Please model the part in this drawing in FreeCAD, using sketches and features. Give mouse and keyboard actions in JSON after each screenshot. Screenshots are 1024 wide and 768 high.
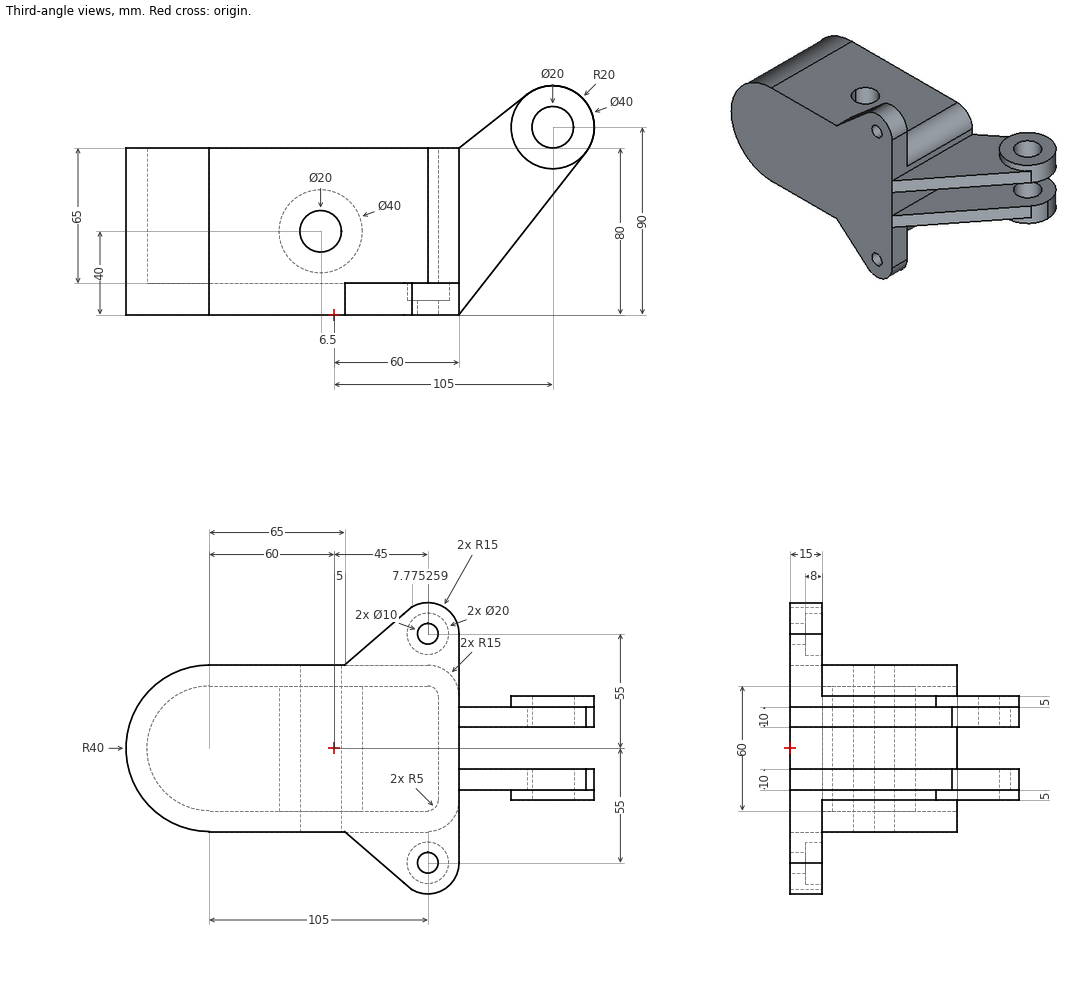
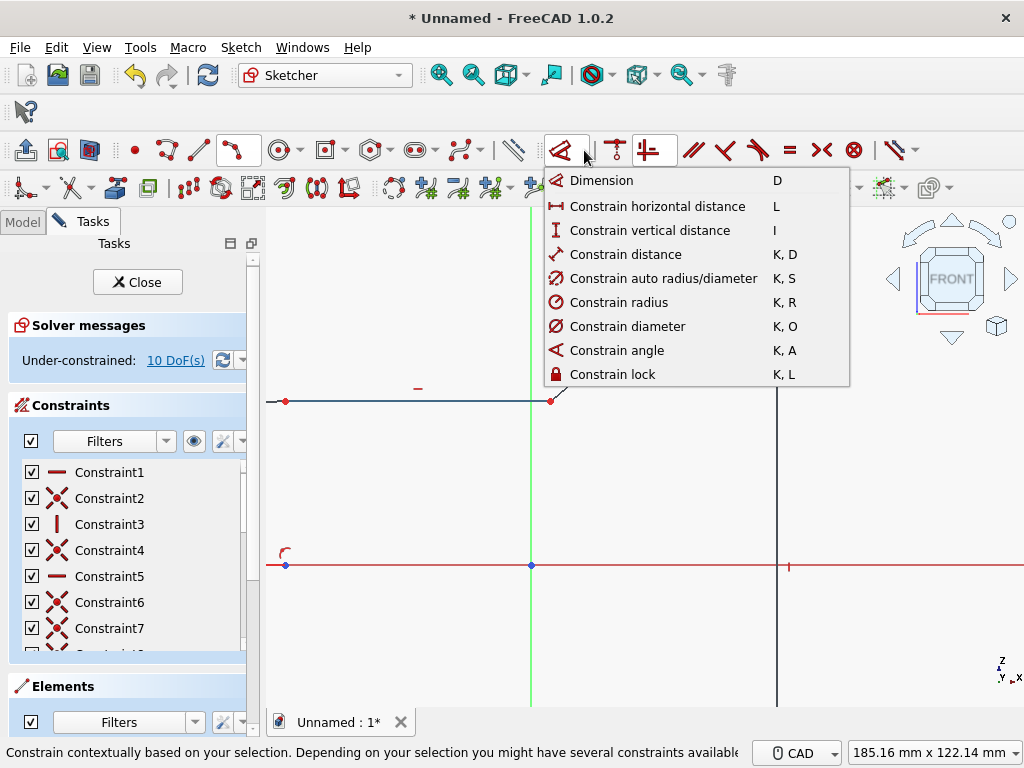
{"action": "left_click", "coordinate": [697, 206]}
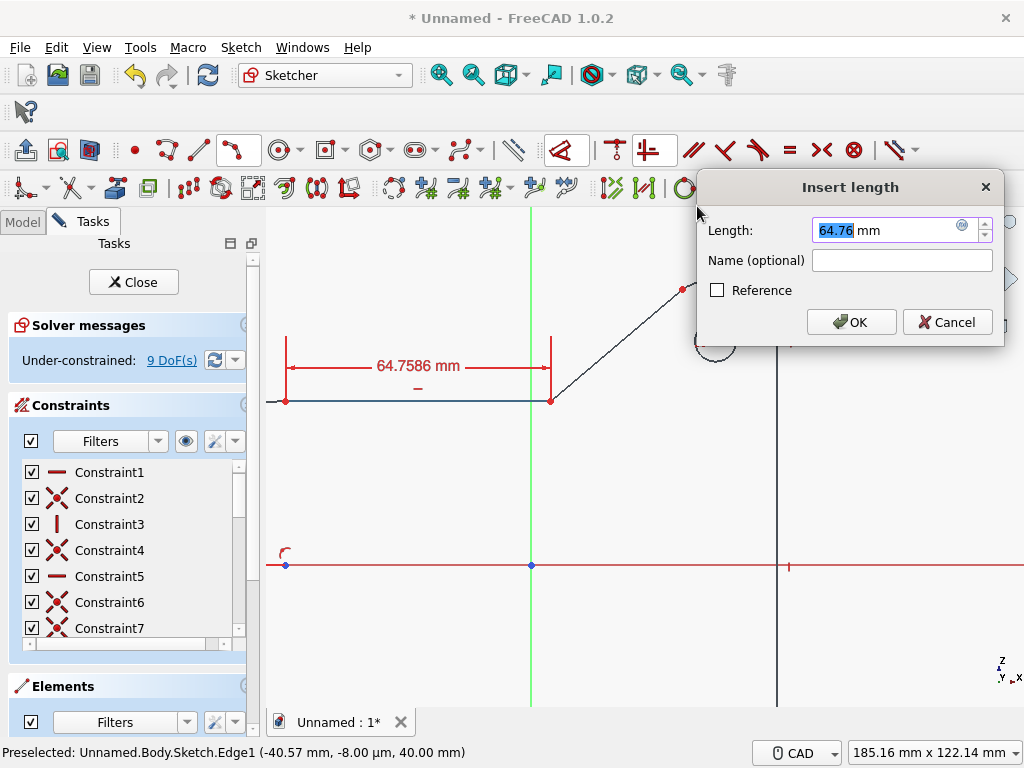
{"action": "type", "text": "65"}
{"action": "key", "text": "Return"}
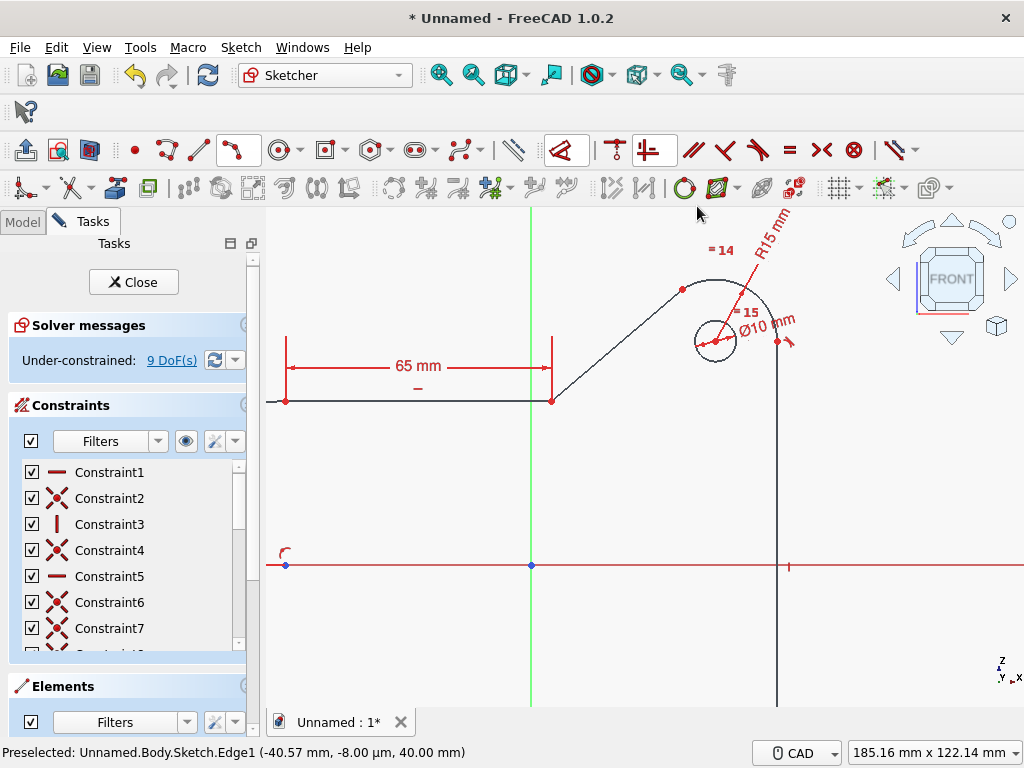
{"action": "scroll", "coordinate": [731, 326], "scroll_direction": "down", "scroll_amount": 3}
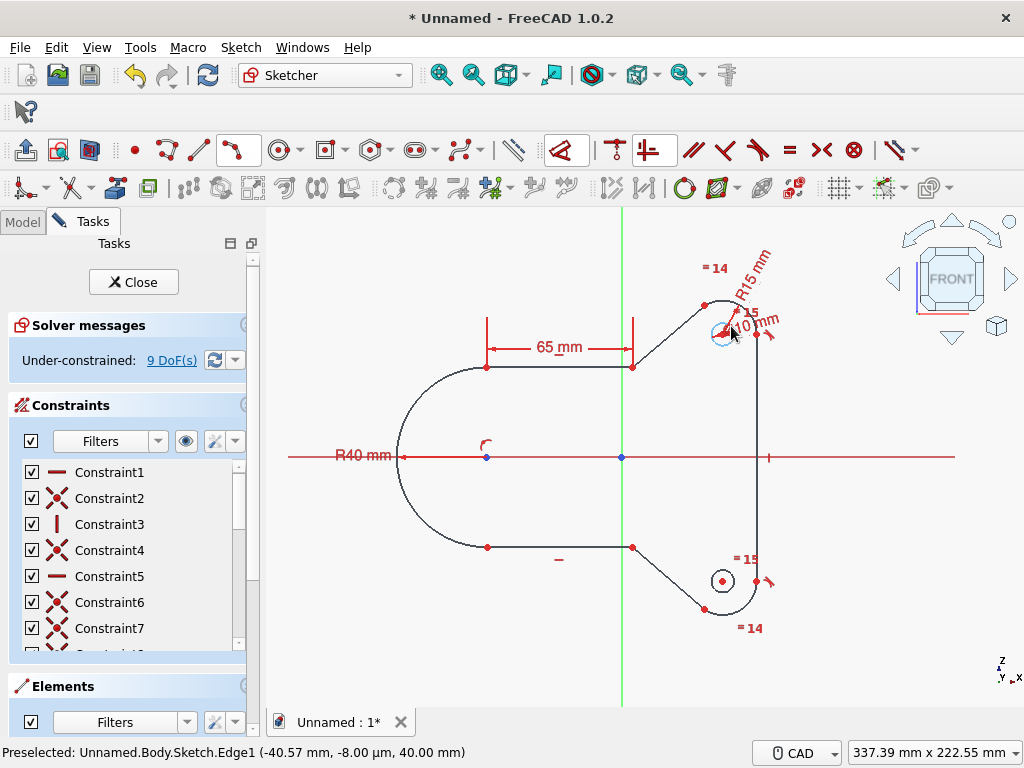
{"action": "left_click", "coordinate": [589, 547]}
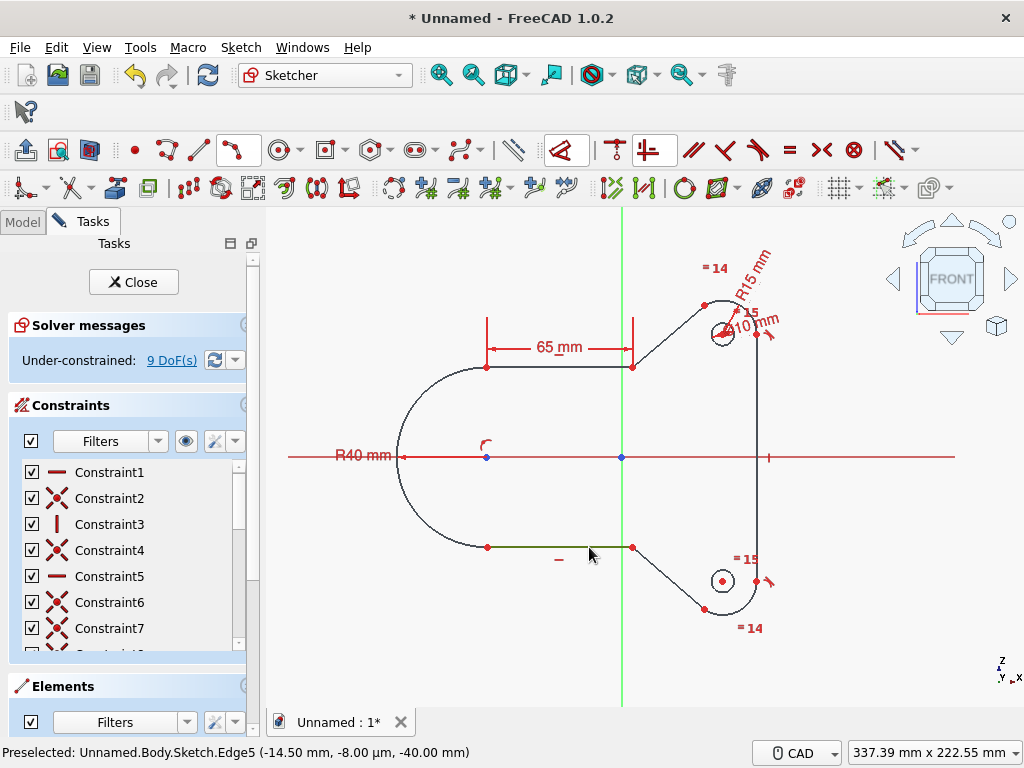
{"action": "key", "text": "l"}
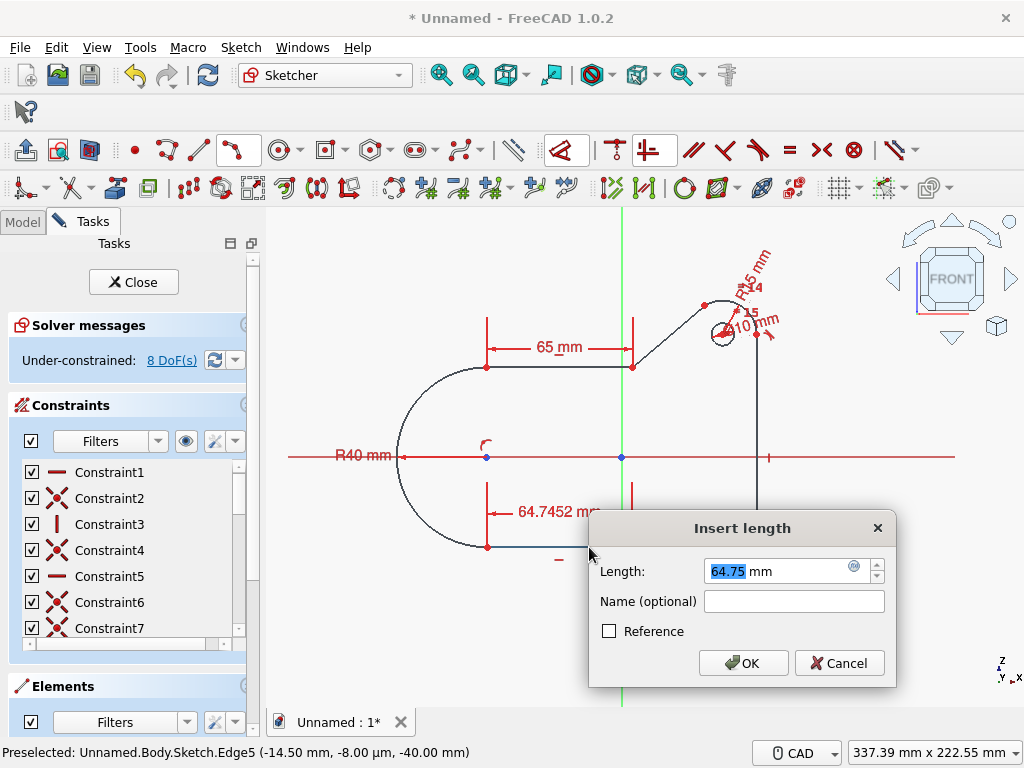
{"action": "type", "text": "65"}
{"action": "key", "text": "Return"}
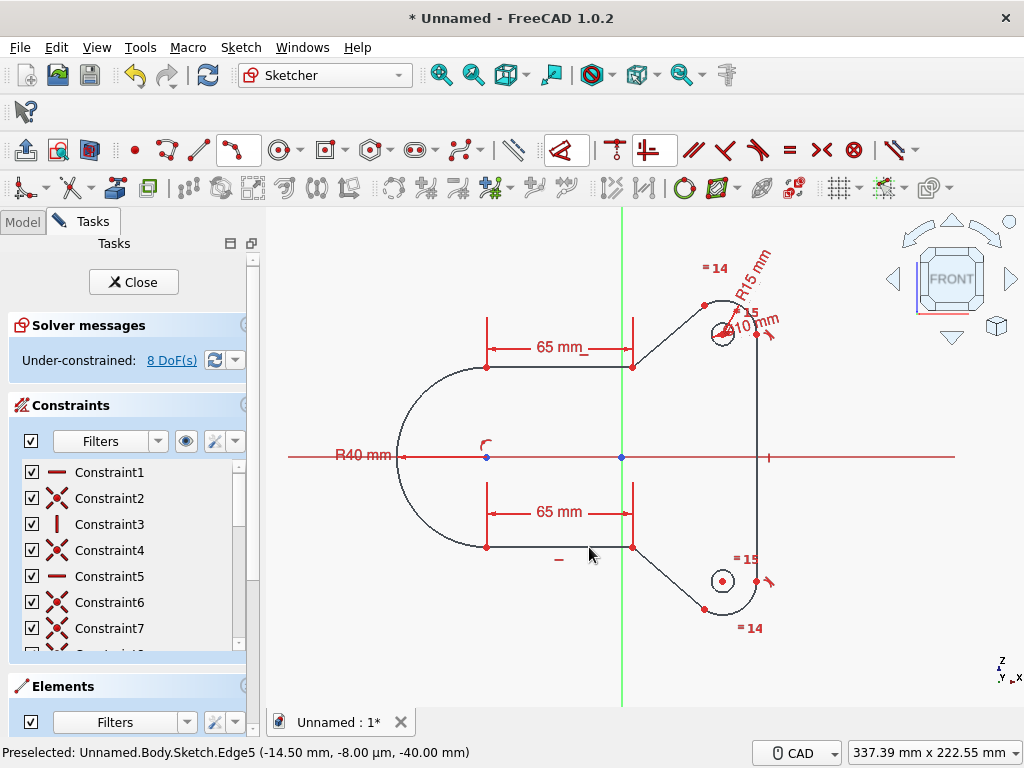
{"action": "scroll", "coordinate": [633, 367], "scroll_direction": "up", "scroll_amount": 7}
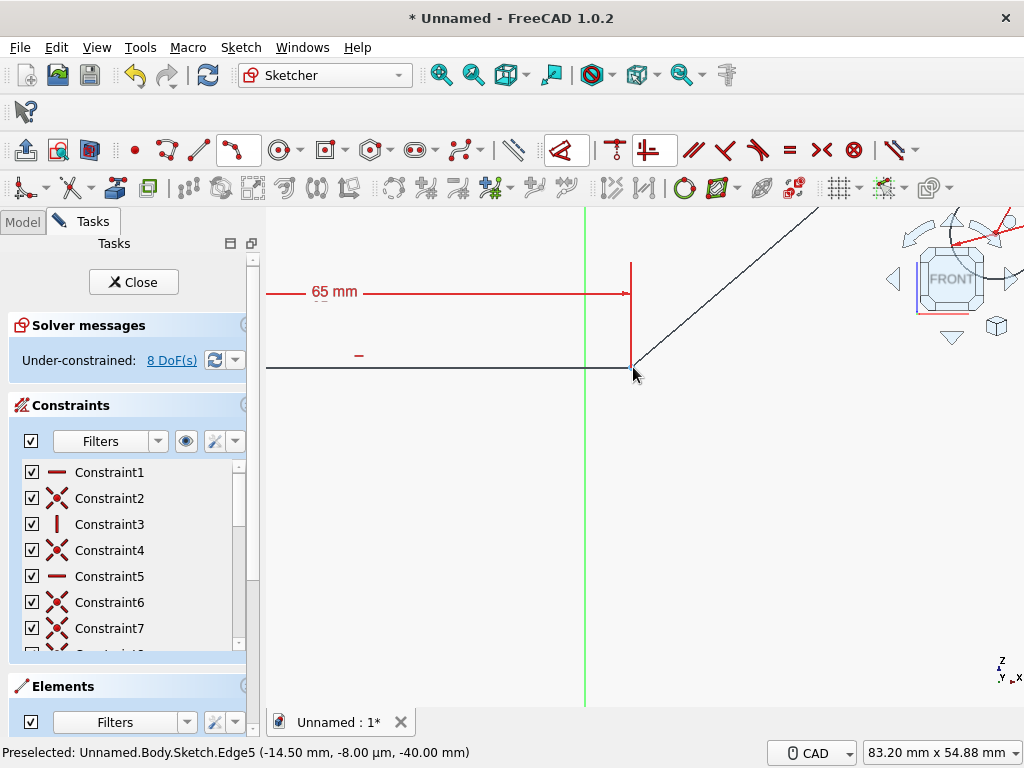
{"action": "left_click", "coordinate": [631, 368]}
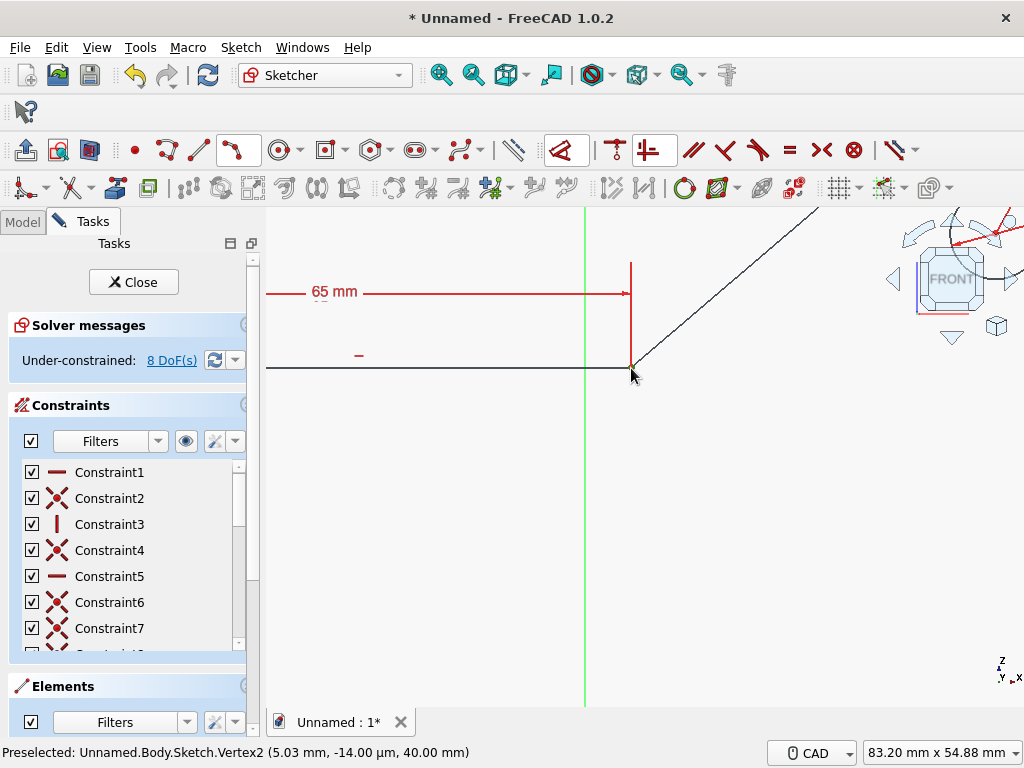
{"action": "left_click", "coordinate": [584, 150]}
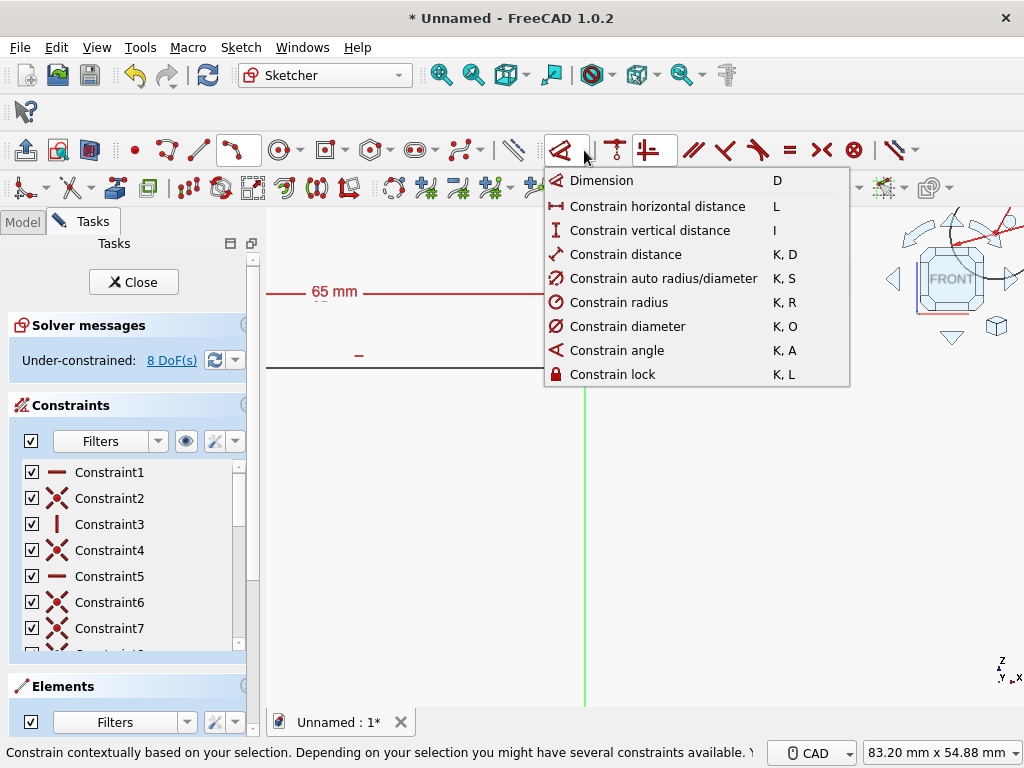
{"action": "left_click", "coordinate": [697, 206]}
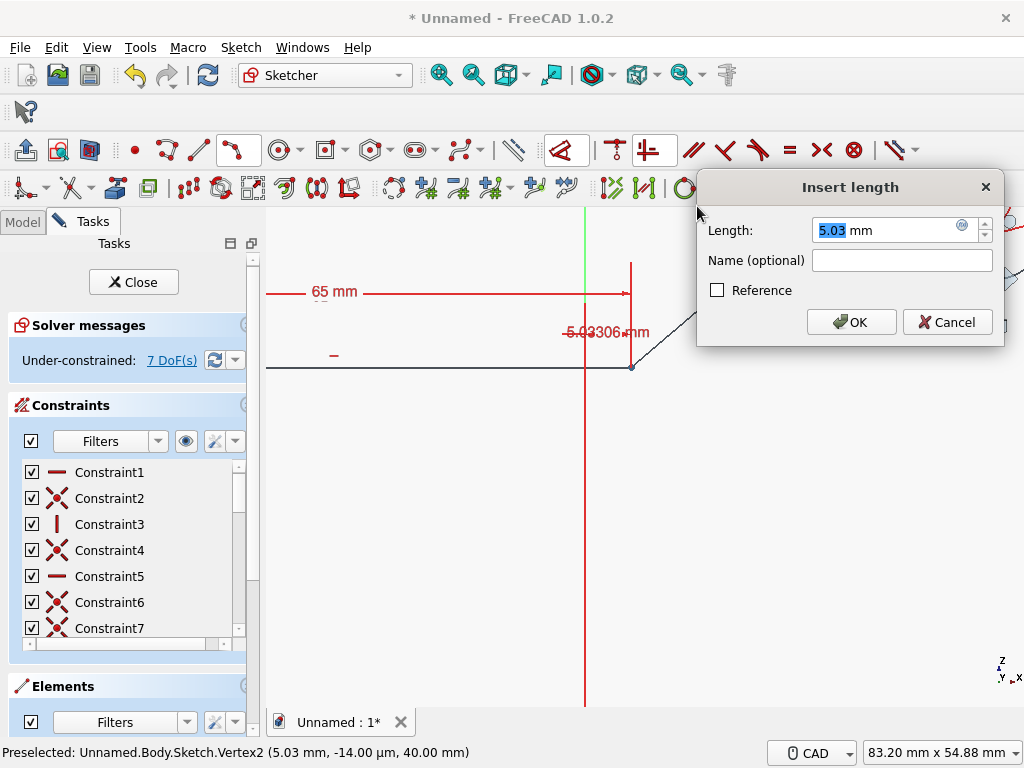
{"action": "type", "text": "5"}
{"action": "key", "text": "Return"}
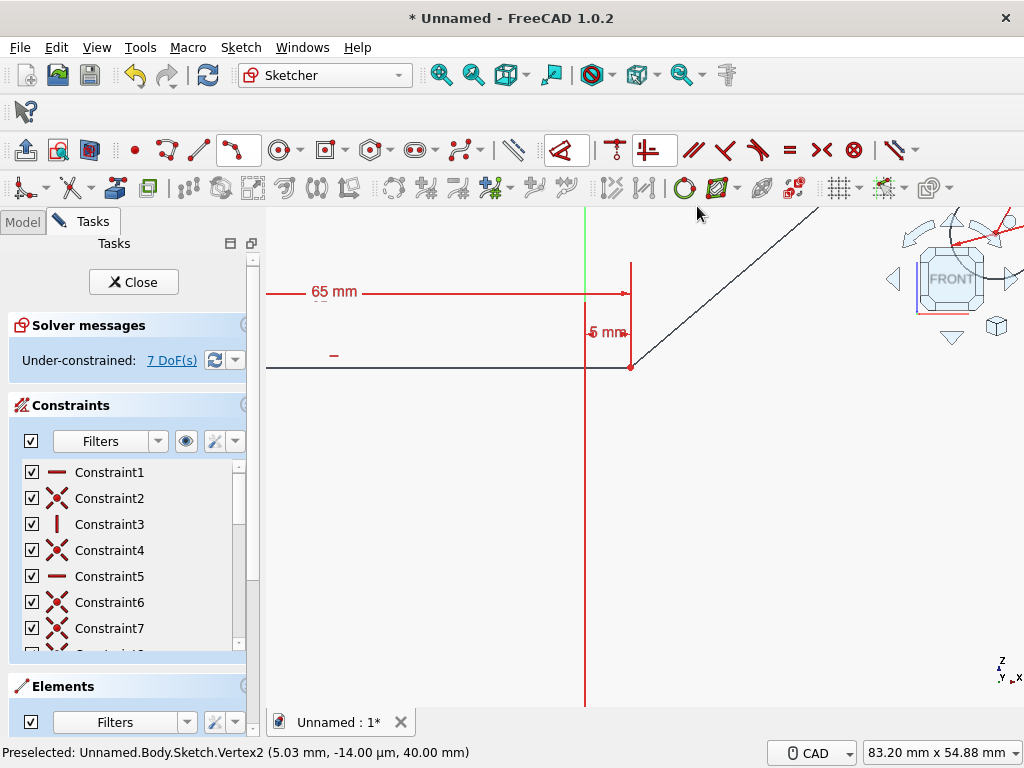
{"action": "scroll", "coordinate": [633, 367], "scroll_direction": "down", "scroll_amount": 7}